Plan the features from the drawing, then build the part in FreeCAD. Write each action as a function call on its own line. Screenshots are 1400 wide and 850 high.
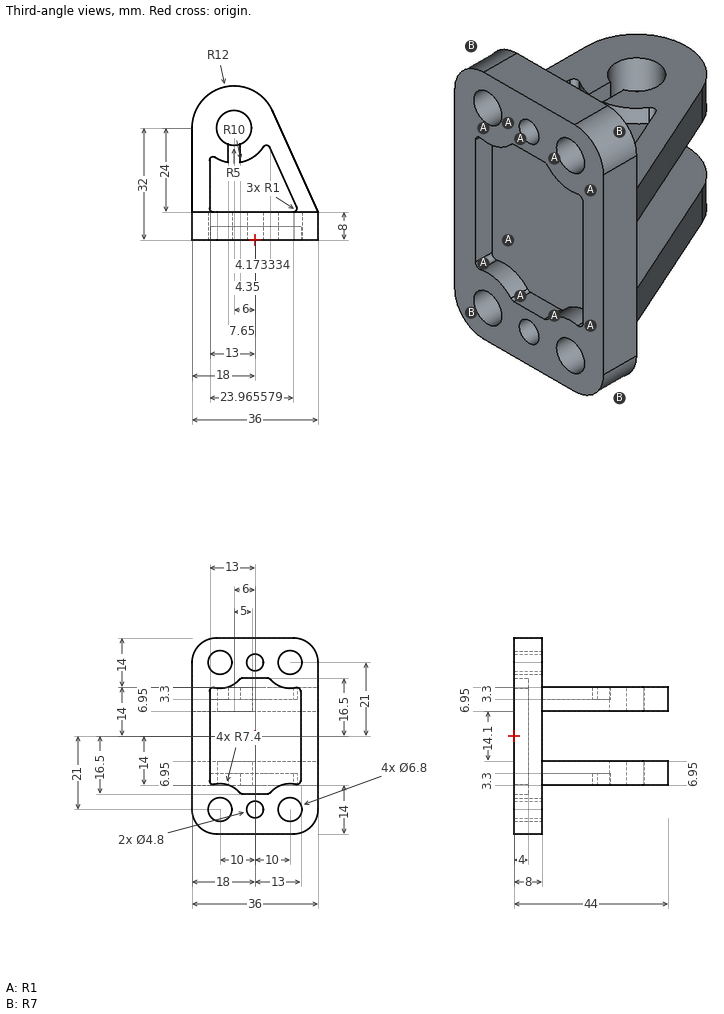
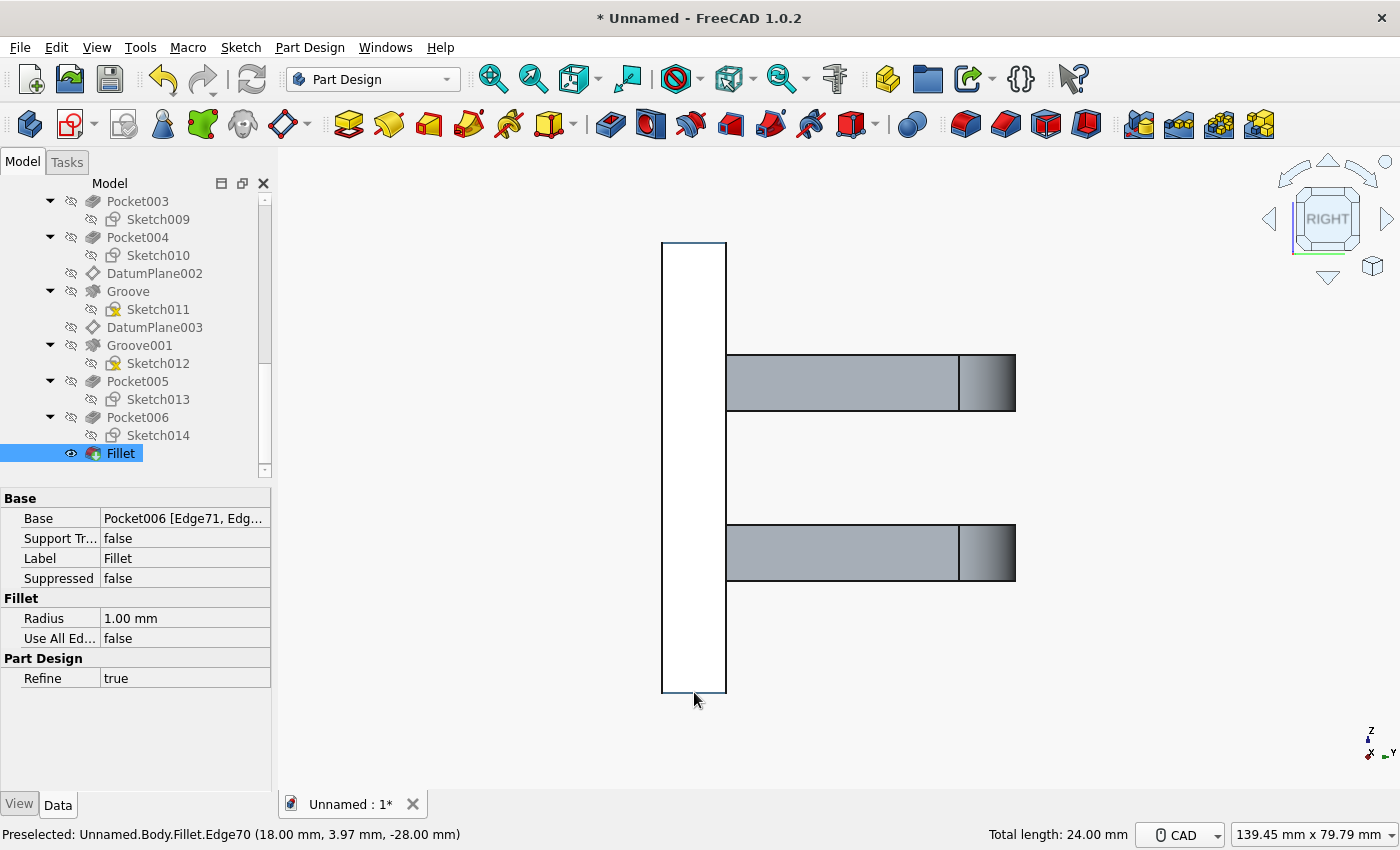
key(5)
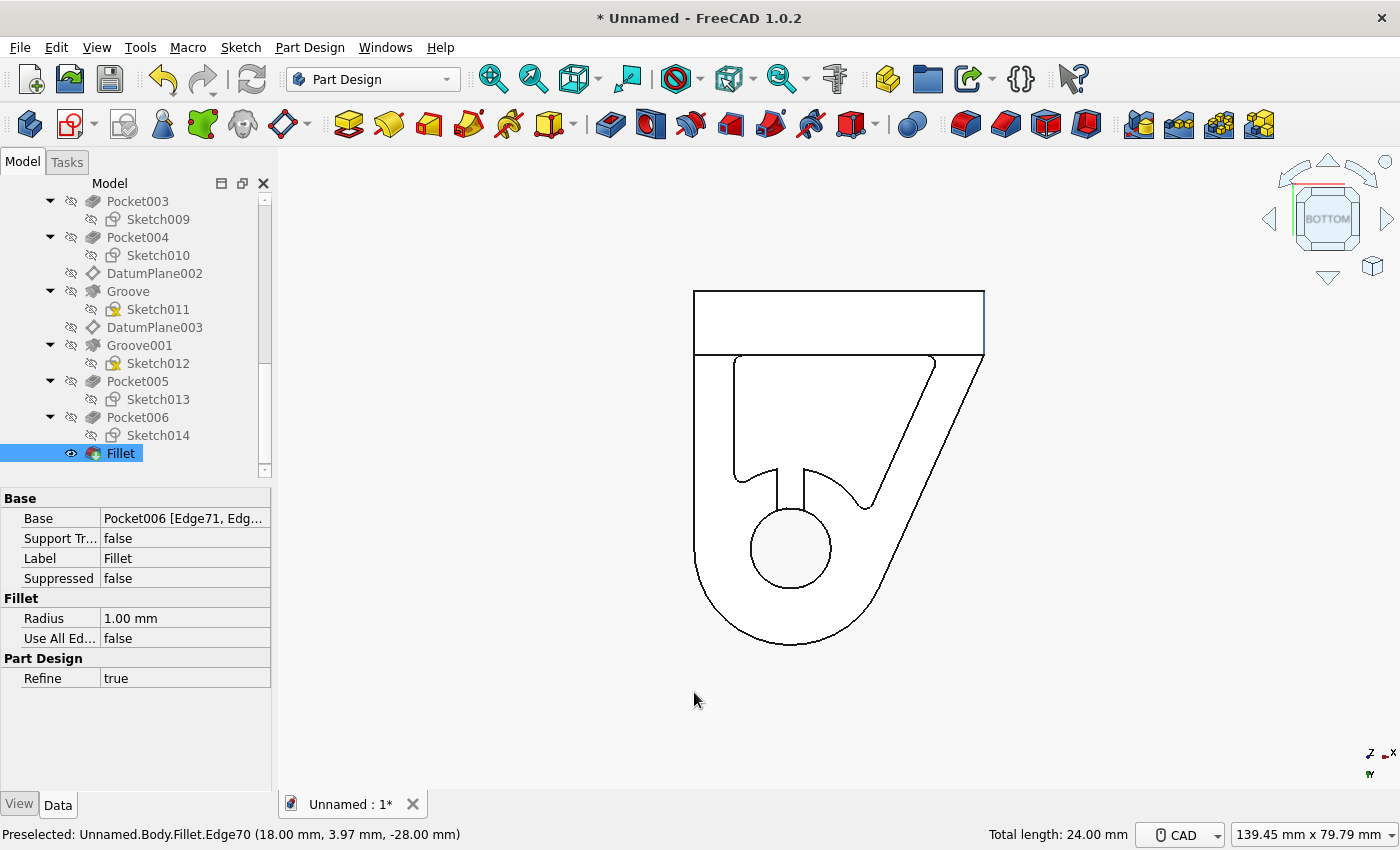
click(694, 322, ctrl)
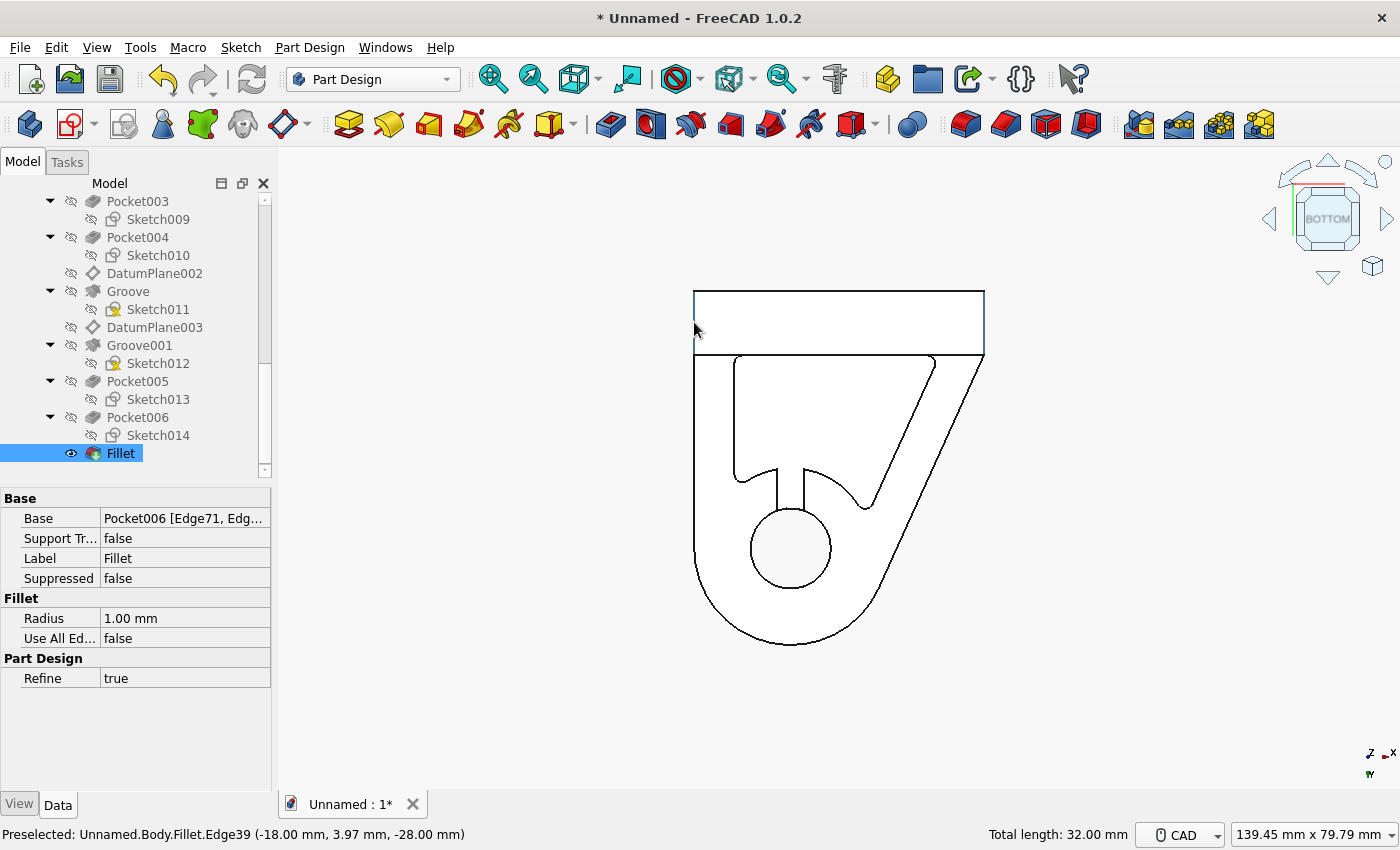
click(966, 124)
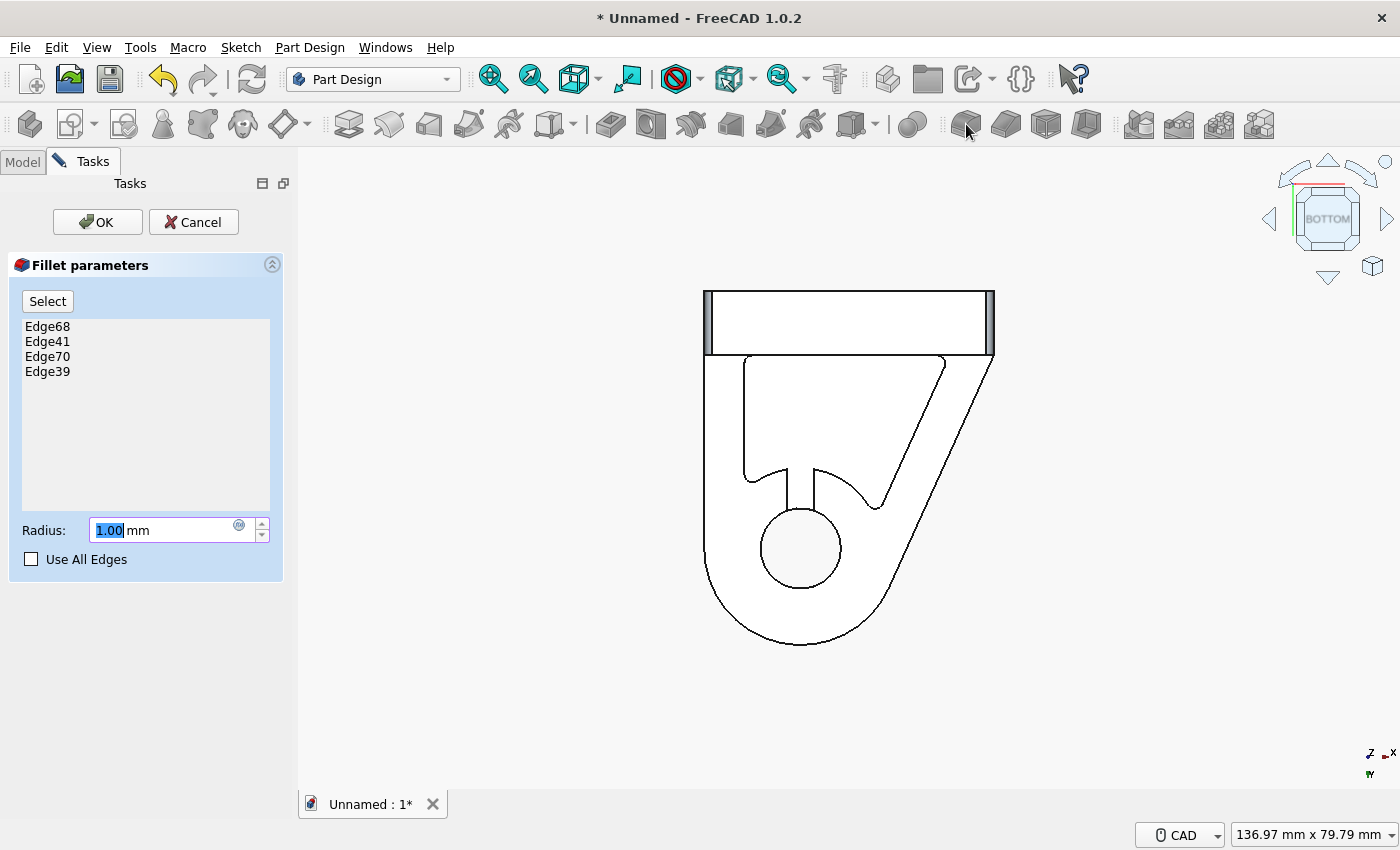
text(7)
key(Tab)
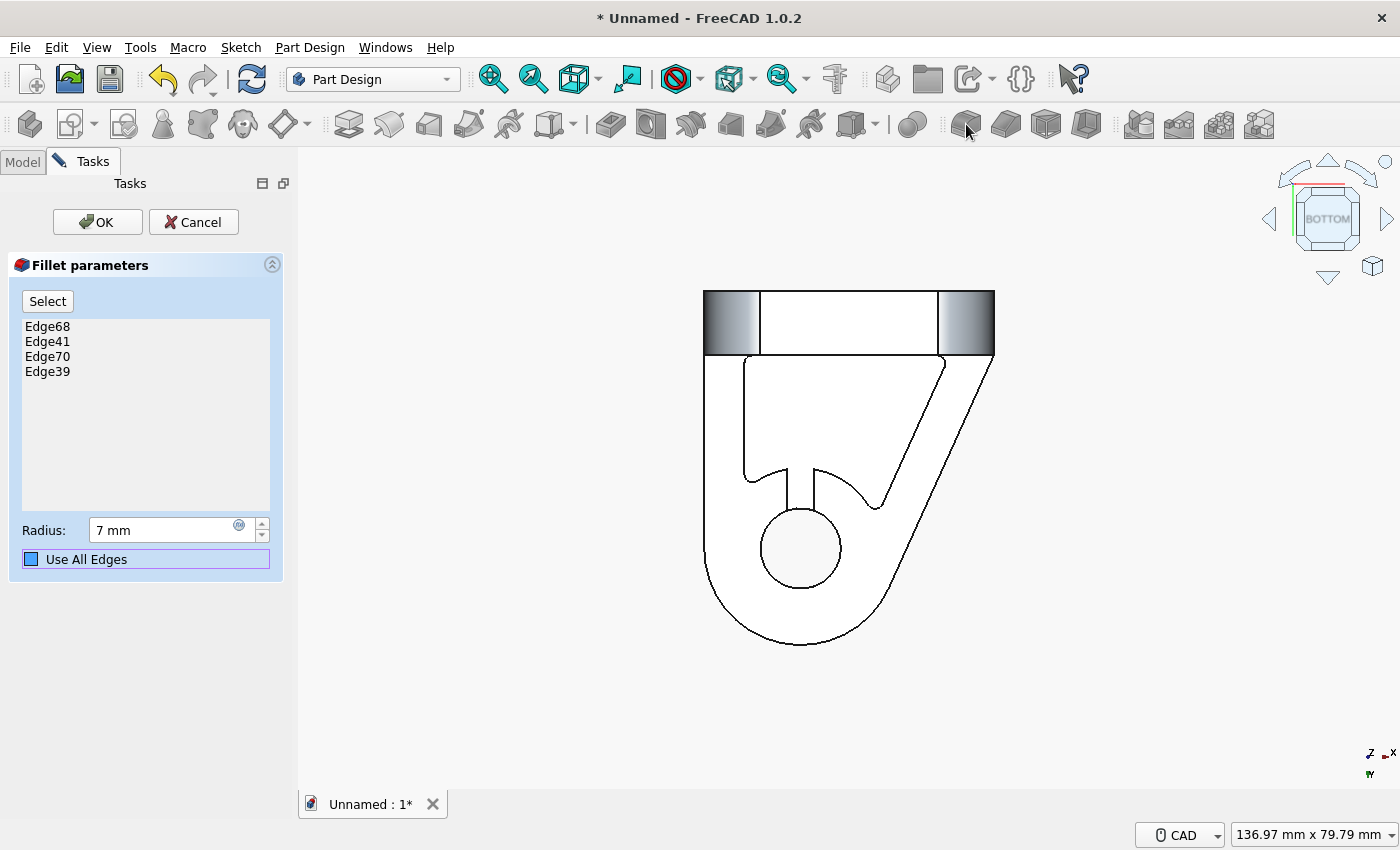
click(98, 222)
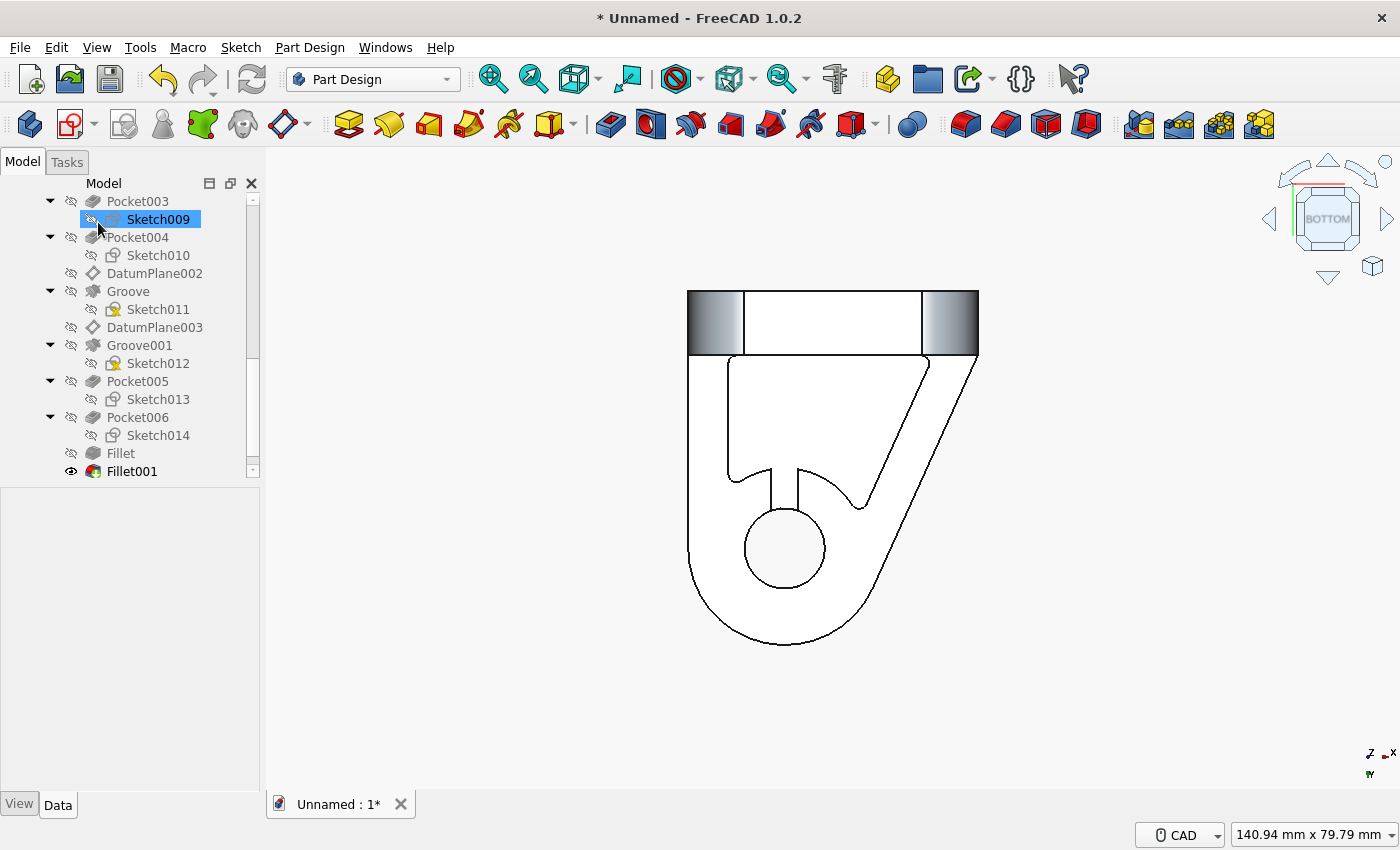
key(0)